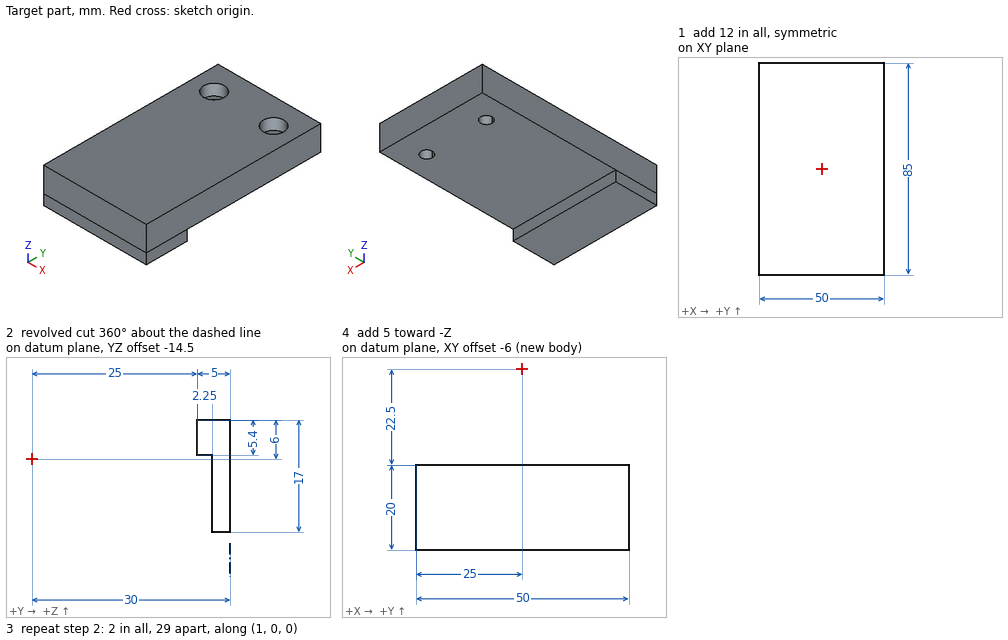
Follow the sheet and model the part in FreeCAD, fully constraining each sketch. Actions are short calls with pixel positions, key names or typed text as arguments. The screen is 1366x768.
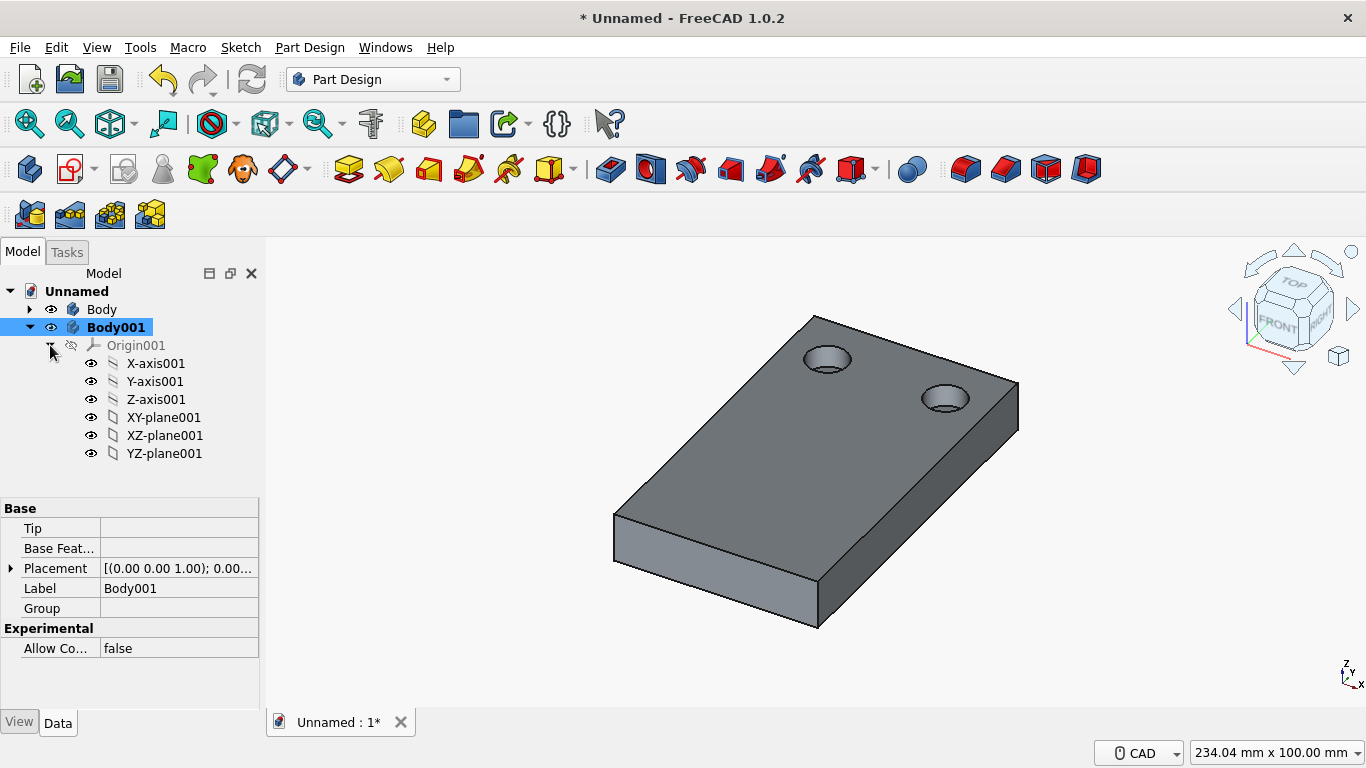
click(136, 417)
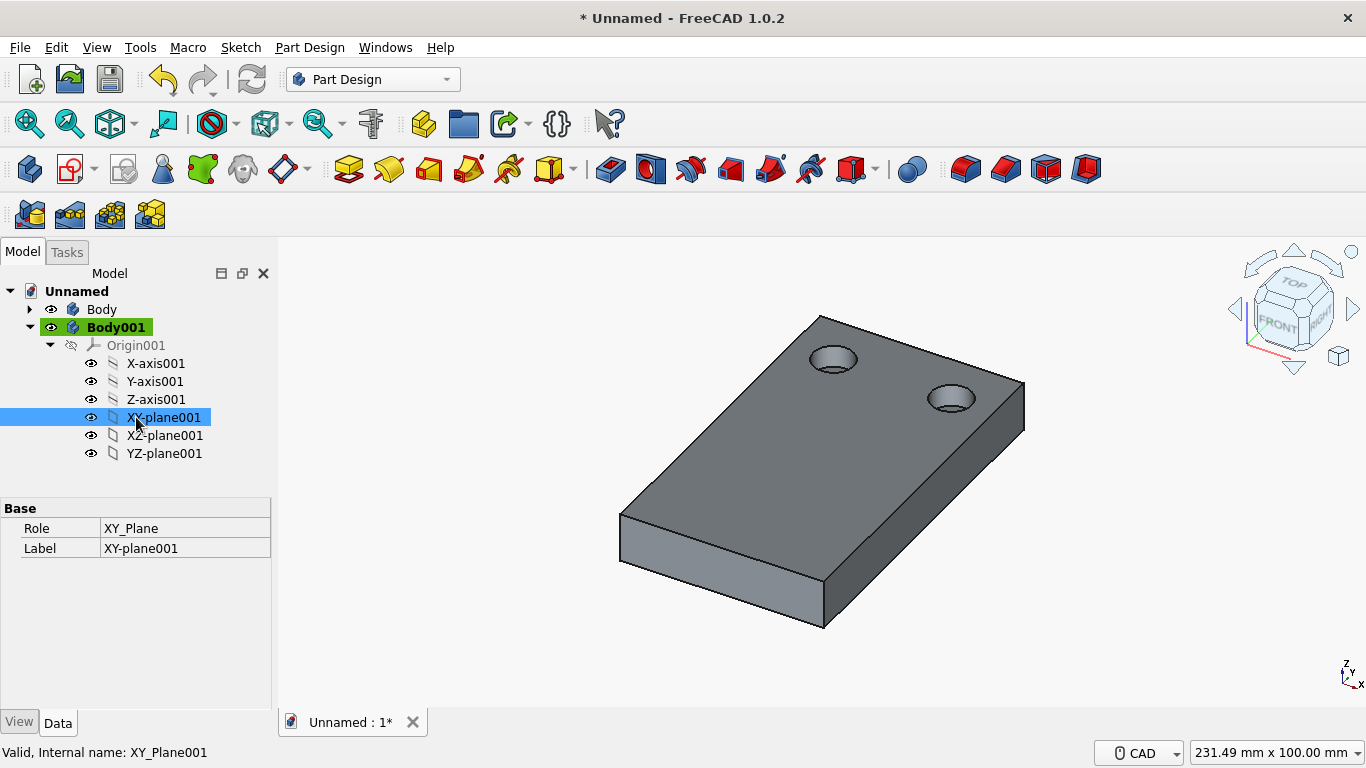
click(284, 170)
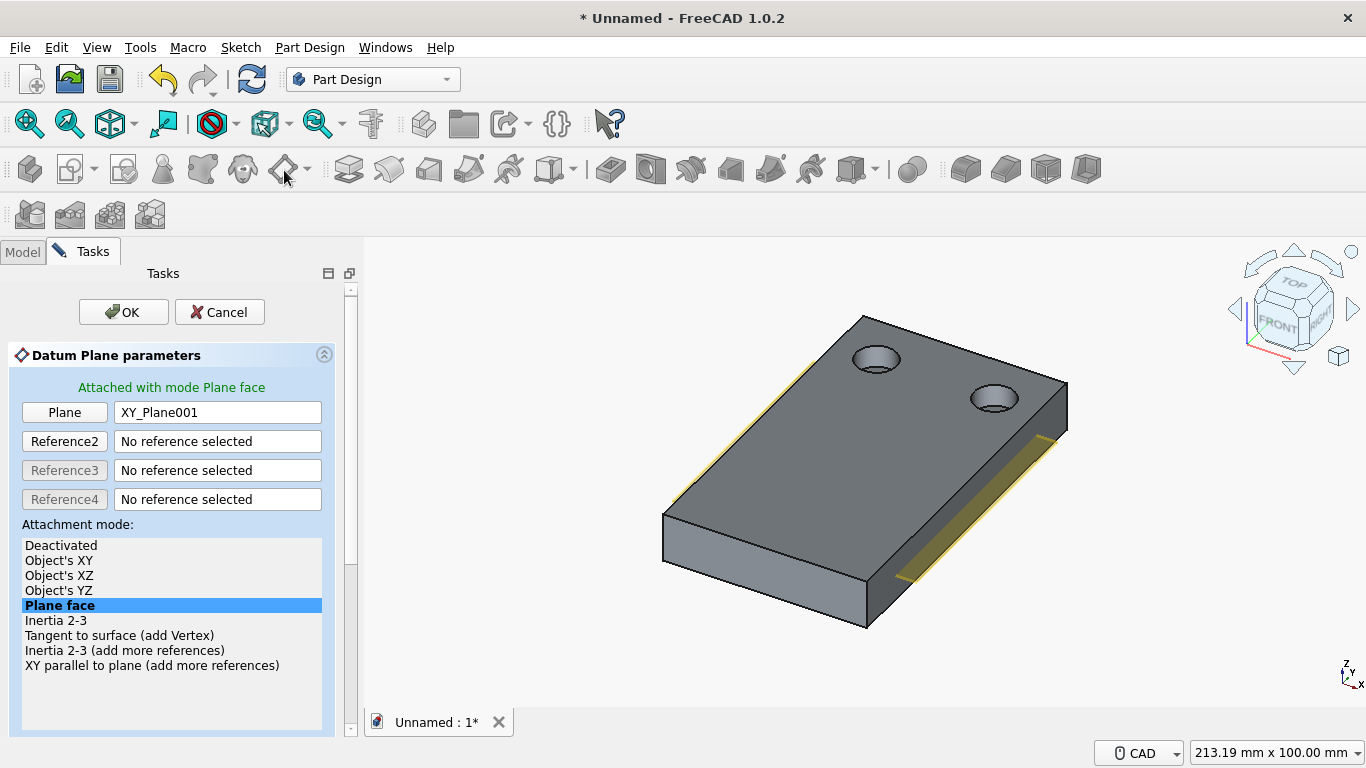
scroll(351, 510, down, 3)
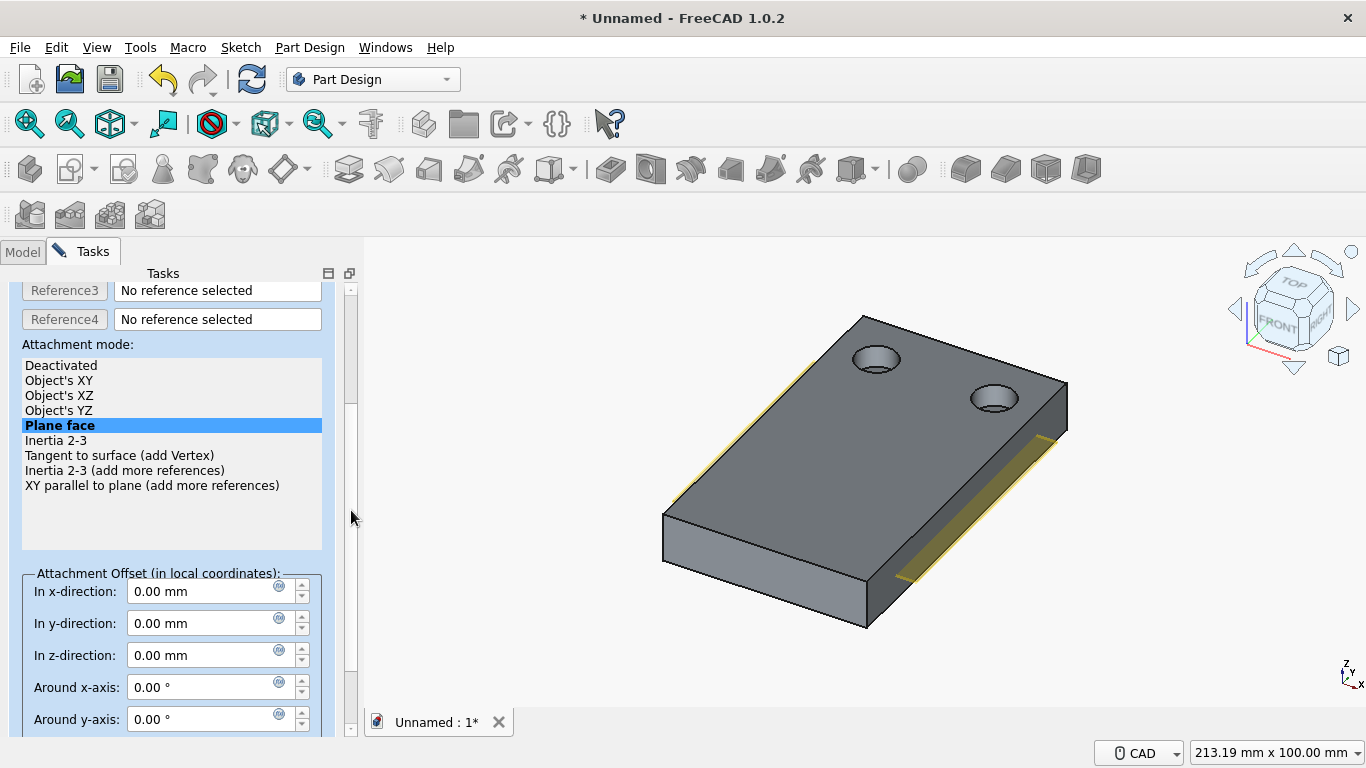
triple_click(210, 655)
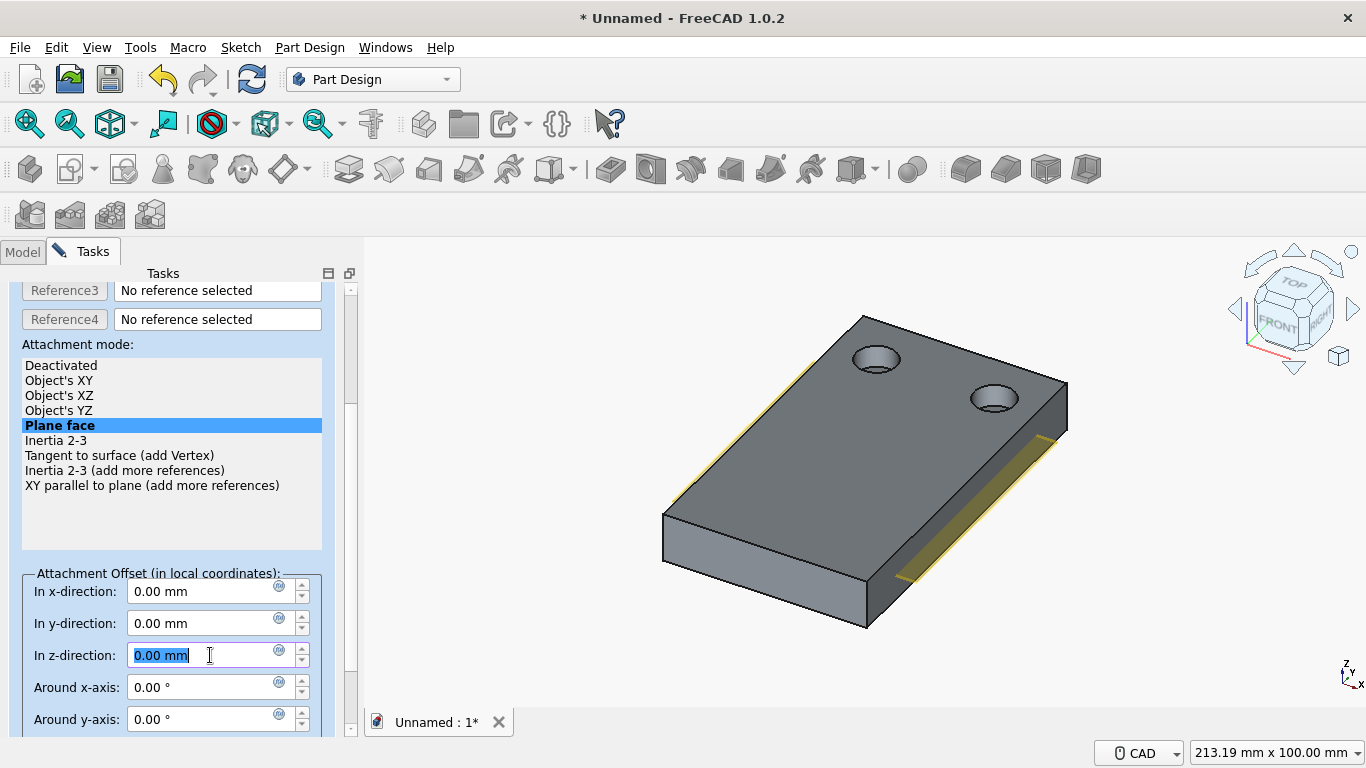
text(-6)
key(Tab)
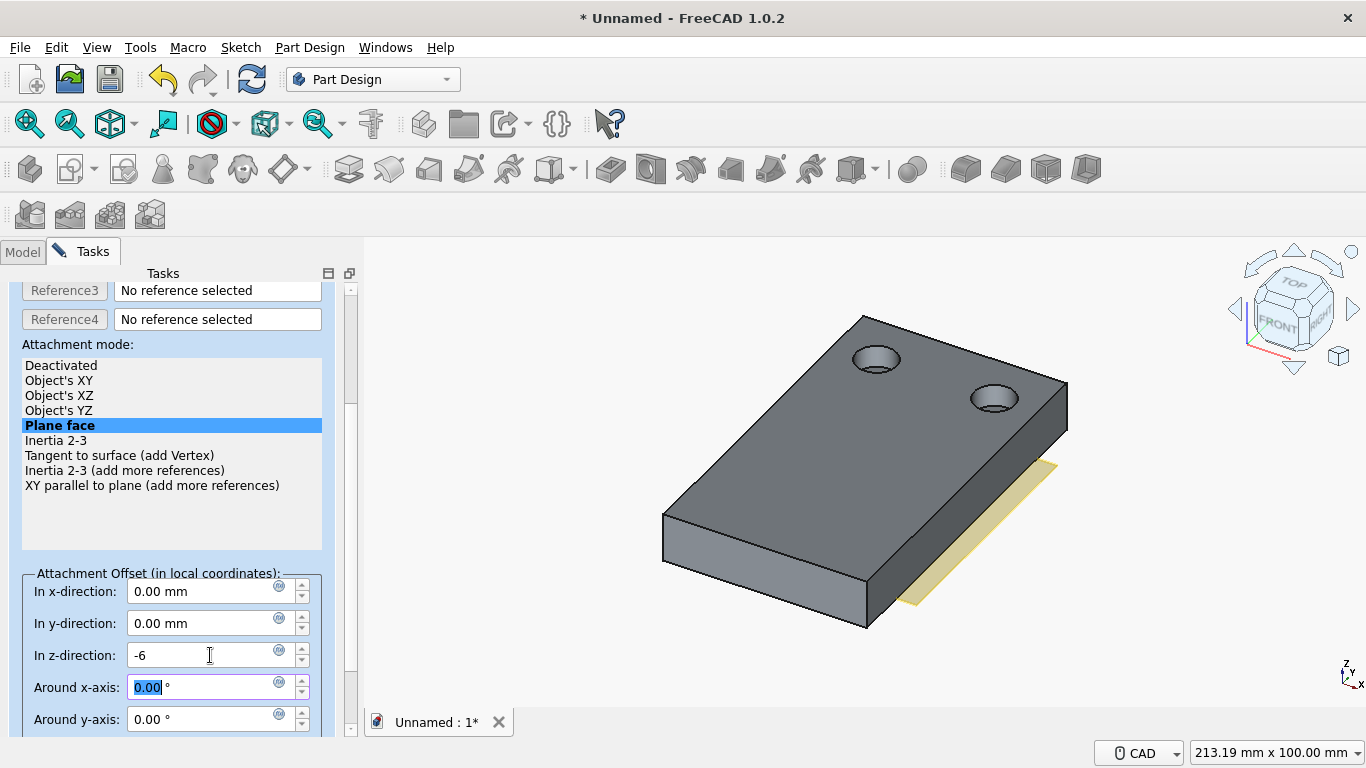
scroll(351, 510, up, 4)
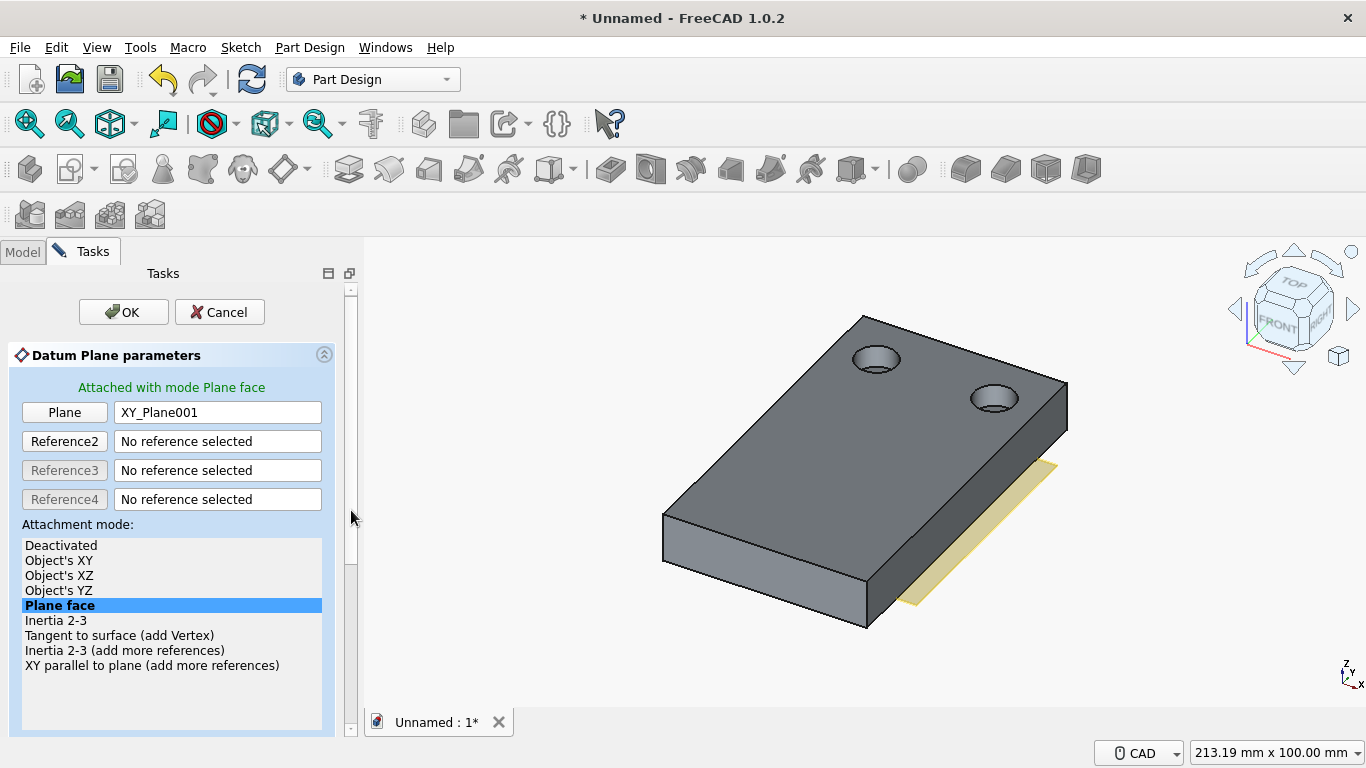
click(124, 312)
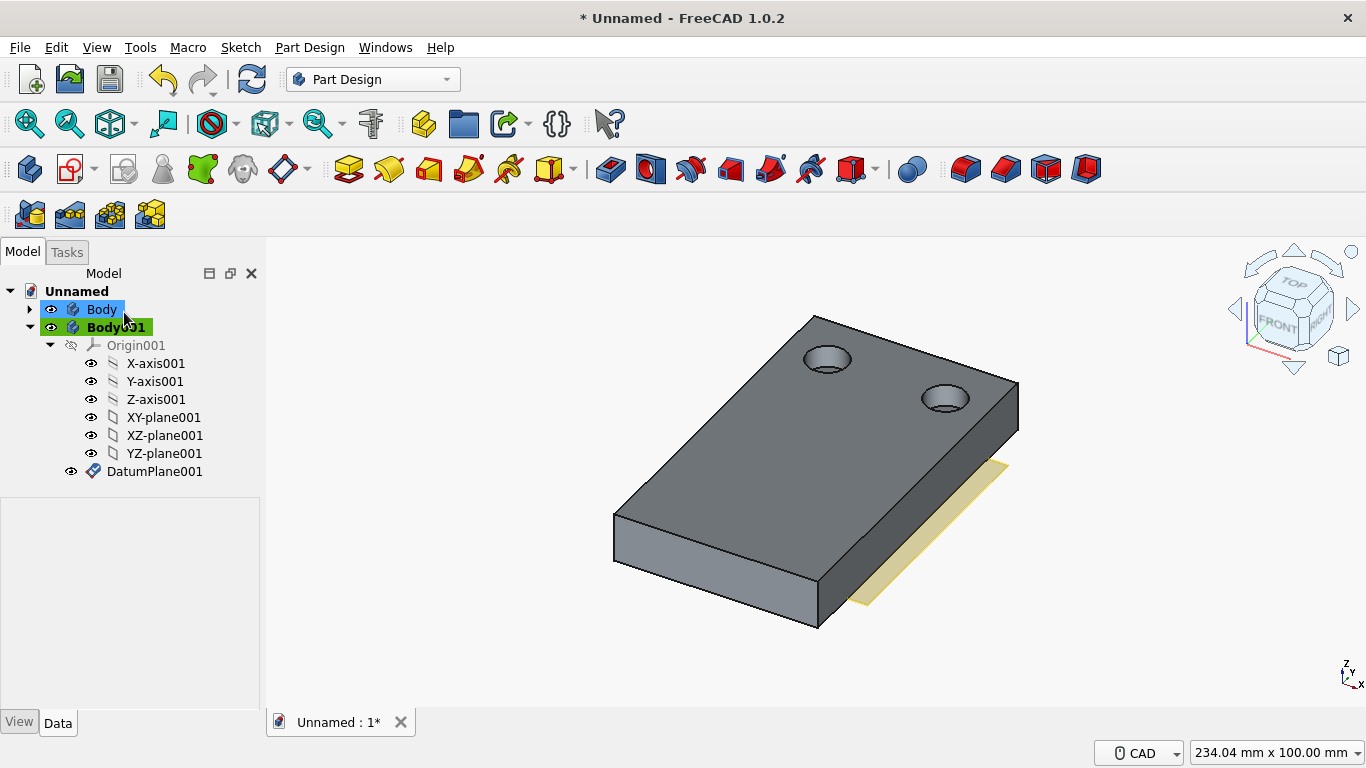
click(116, 471)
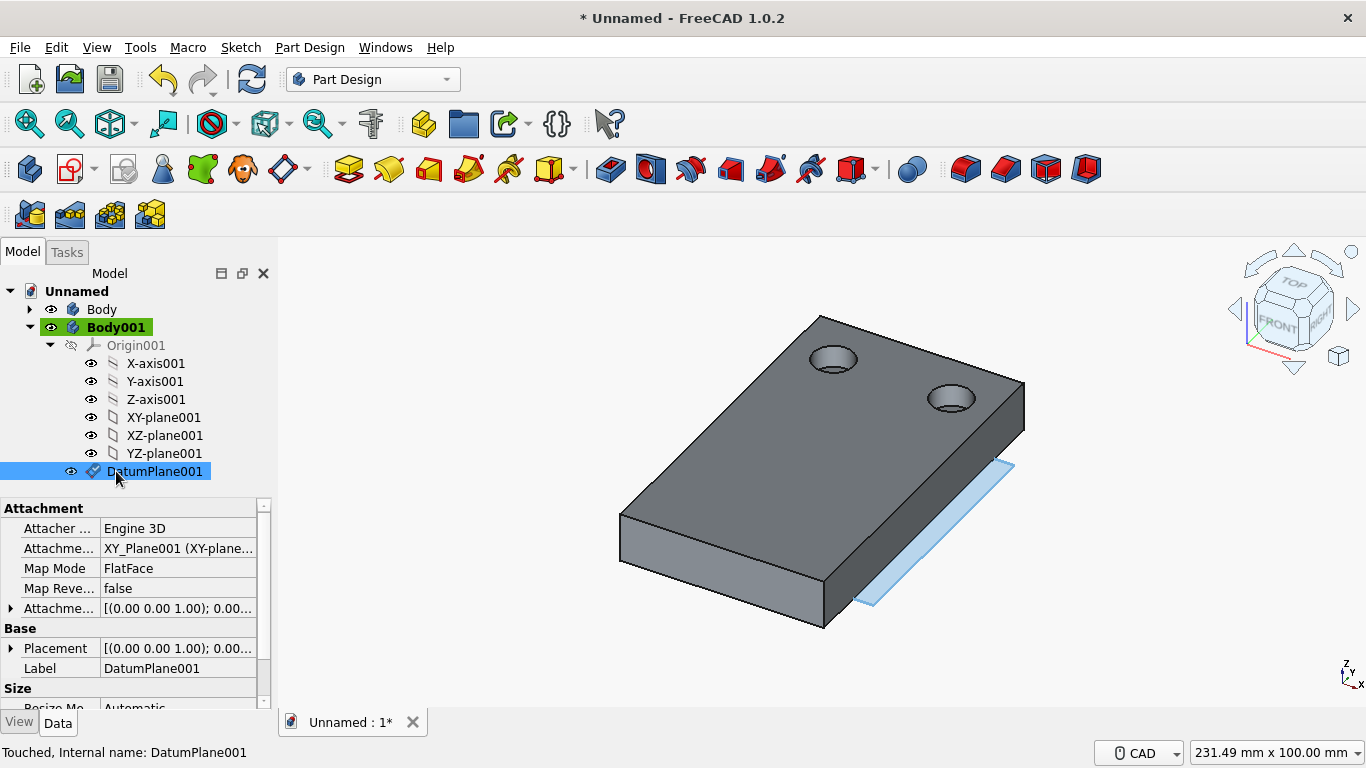
click(70, 170)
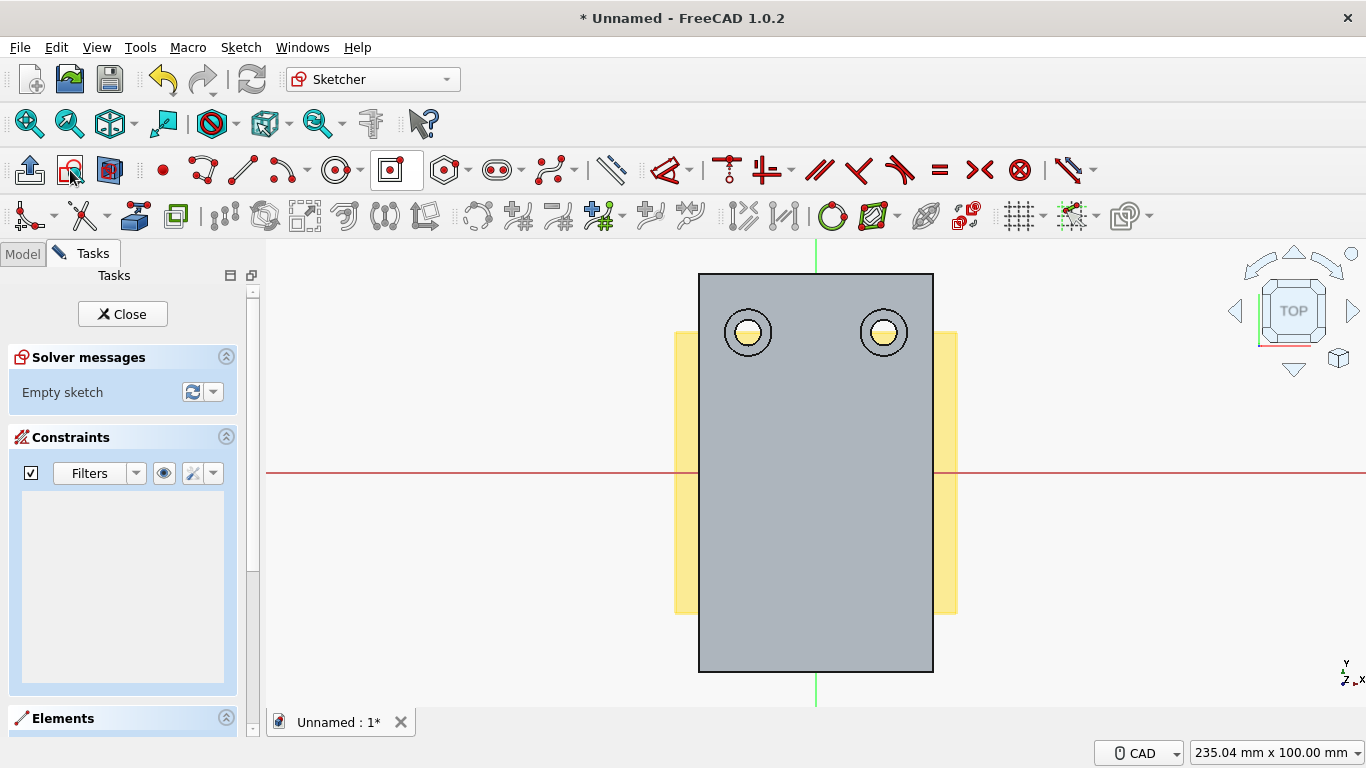
scroll(438, 267, down, 1)